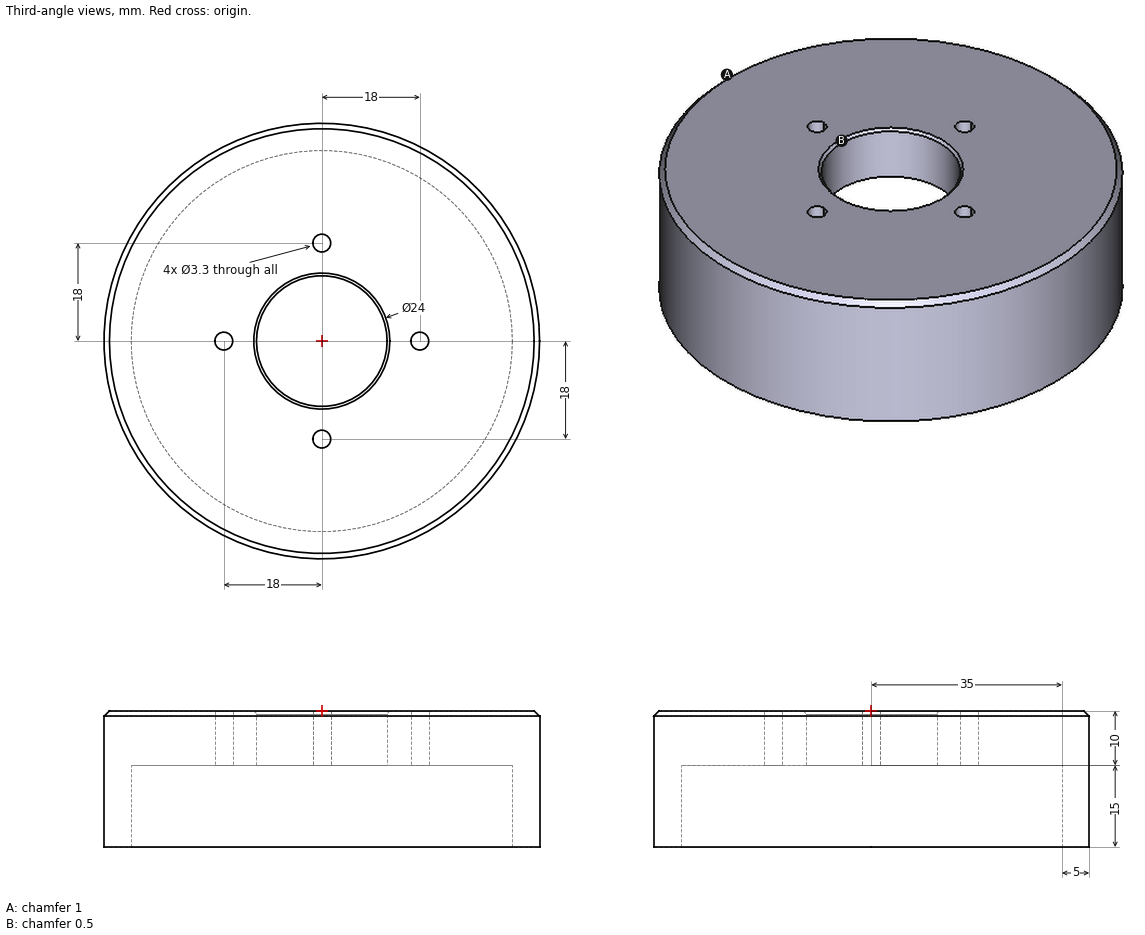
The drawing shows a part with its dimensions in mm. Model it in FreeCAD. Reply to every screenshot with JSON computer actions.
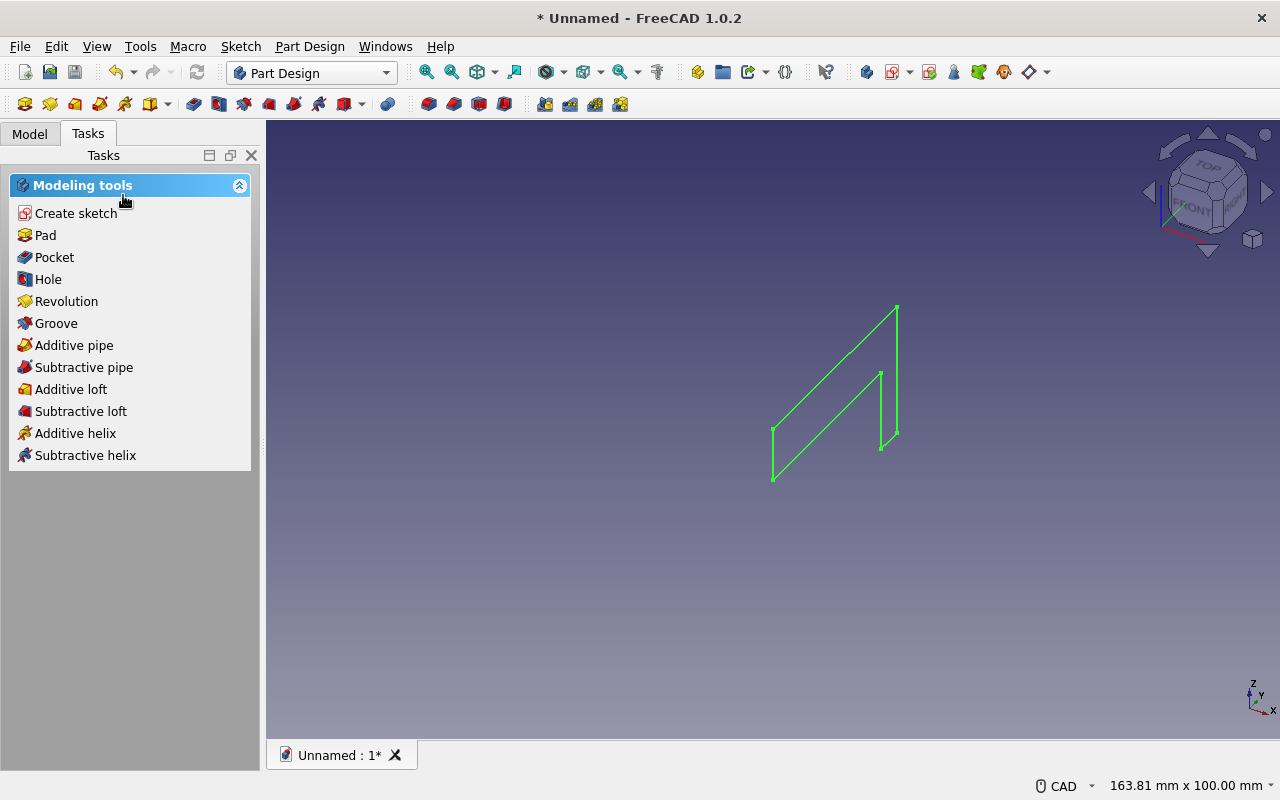
{"action": "left_click", "coordinate": [50, 104]}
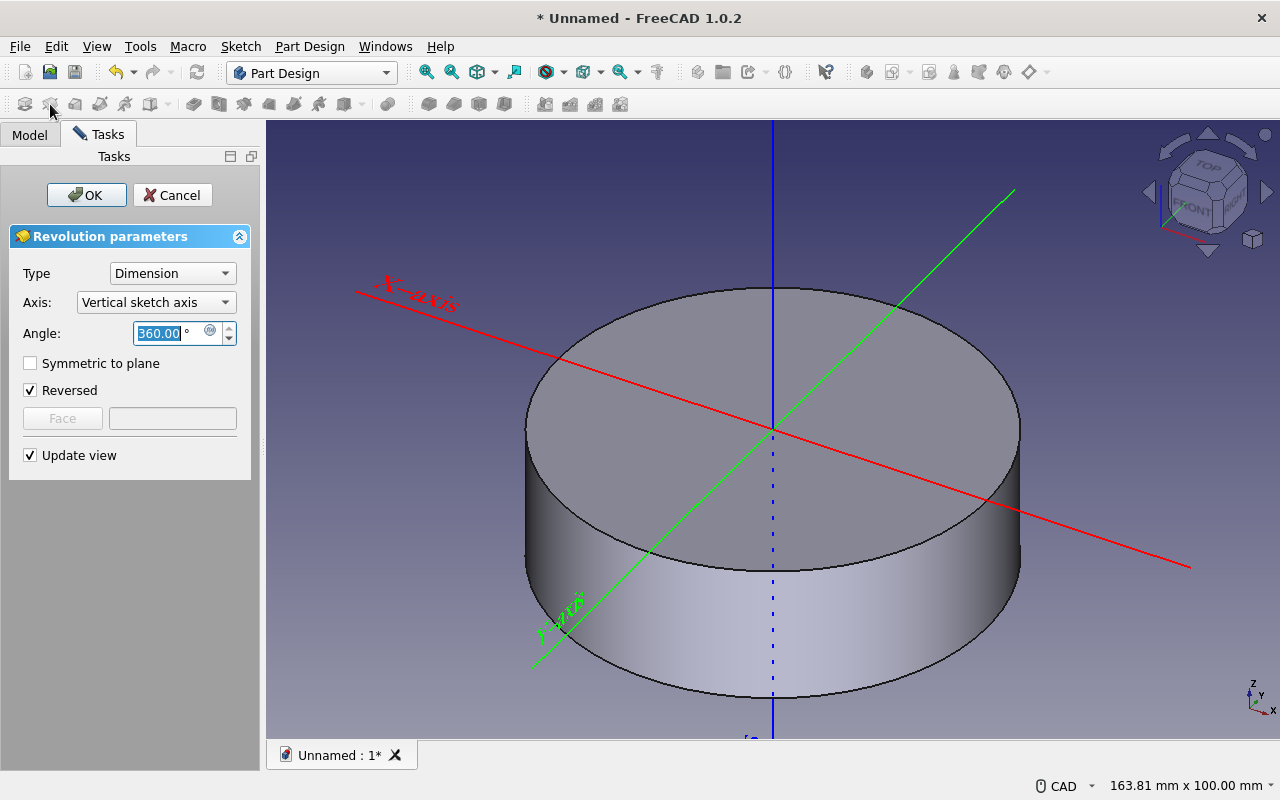
{"action": "left_click", "coordinate": [87, 195]}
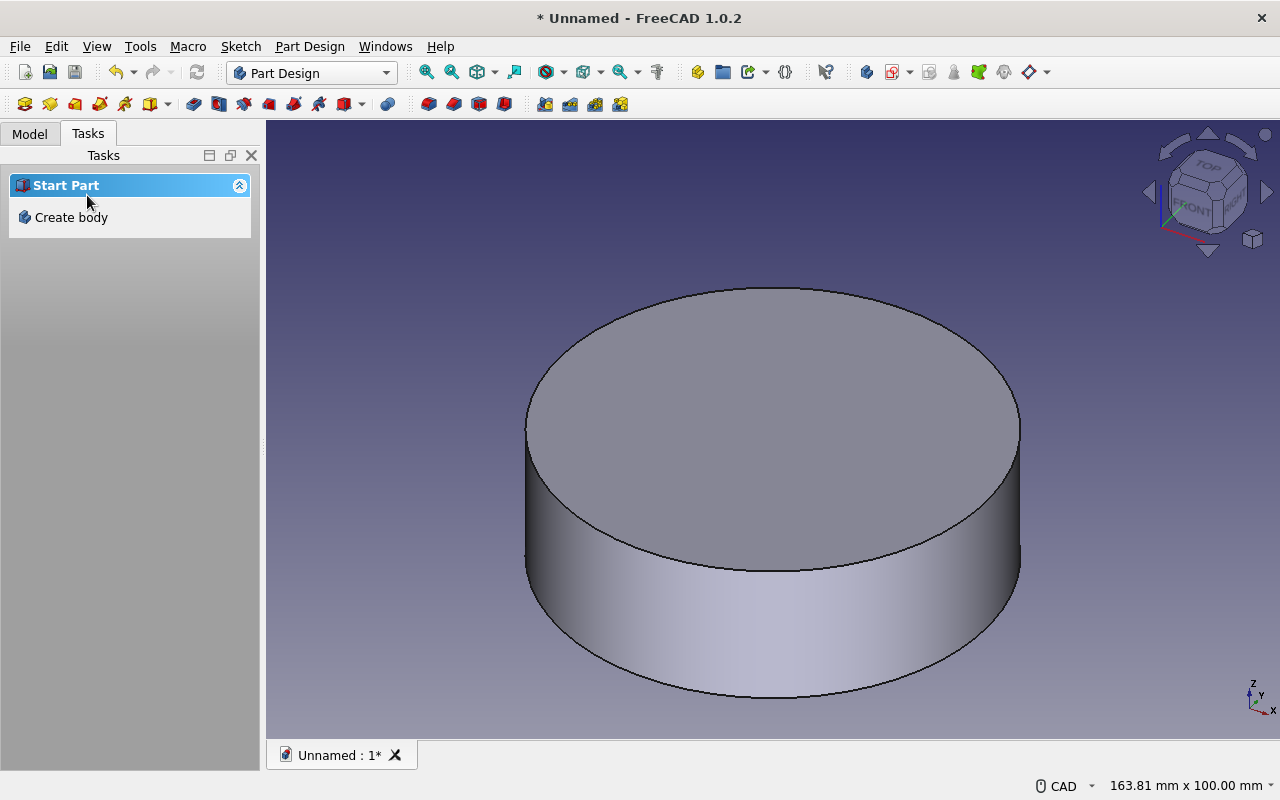
{"action": "key", "text": "v f"}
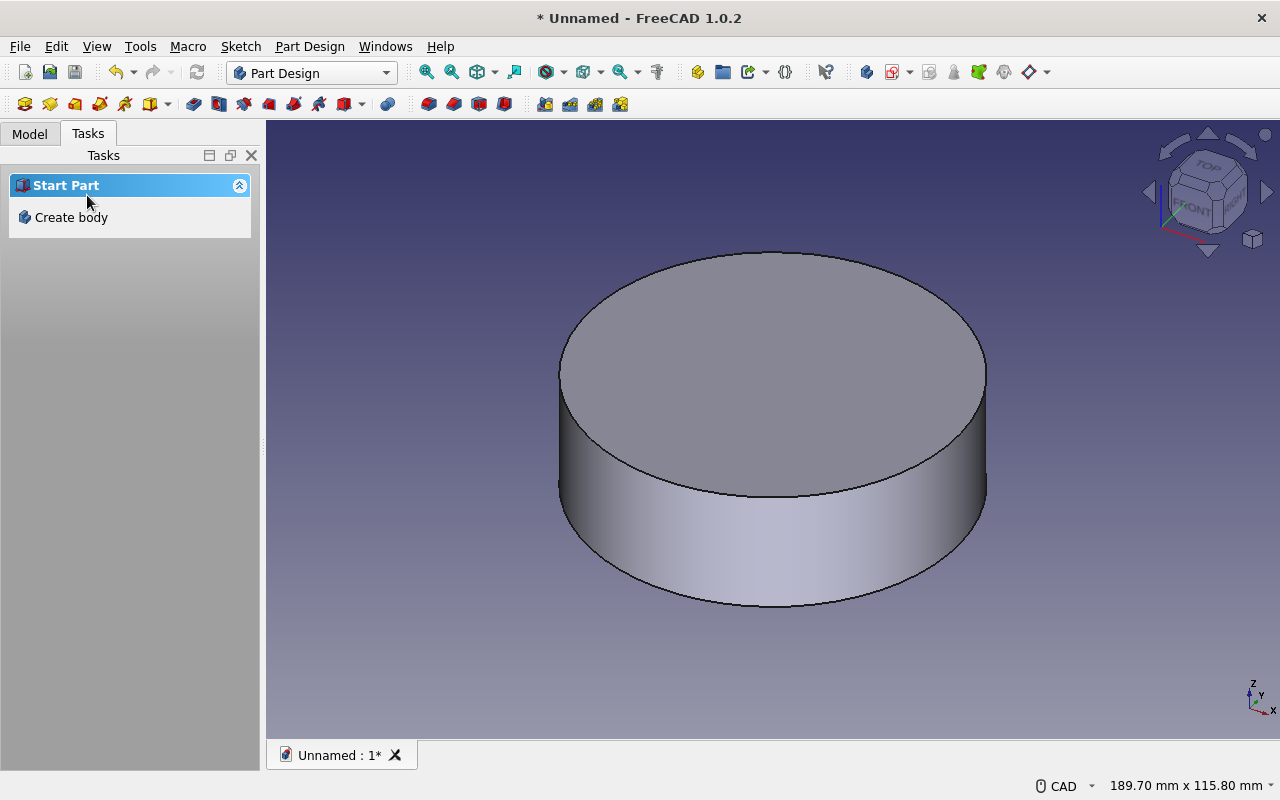
{"action": "left_click", "coordinate": [666, 480]}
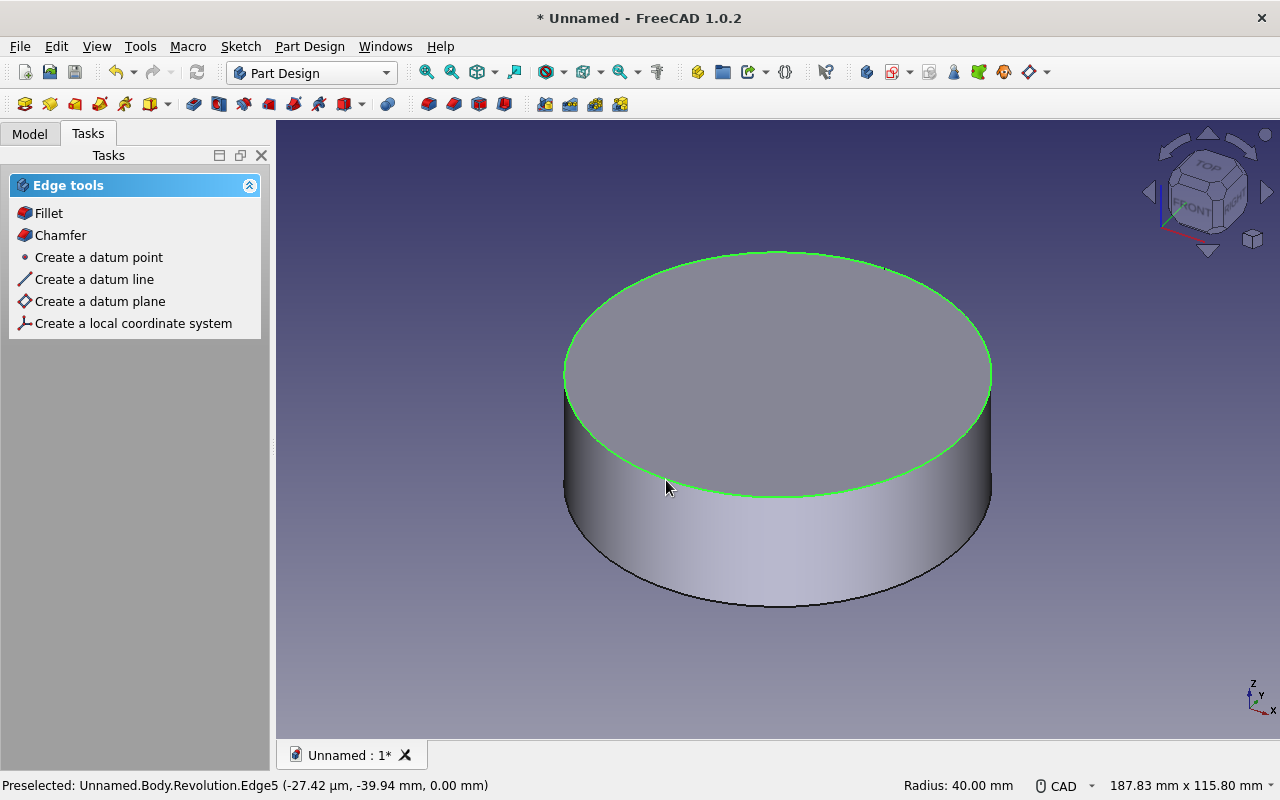
{"action": "left_click", "coordinate": [454, 104]}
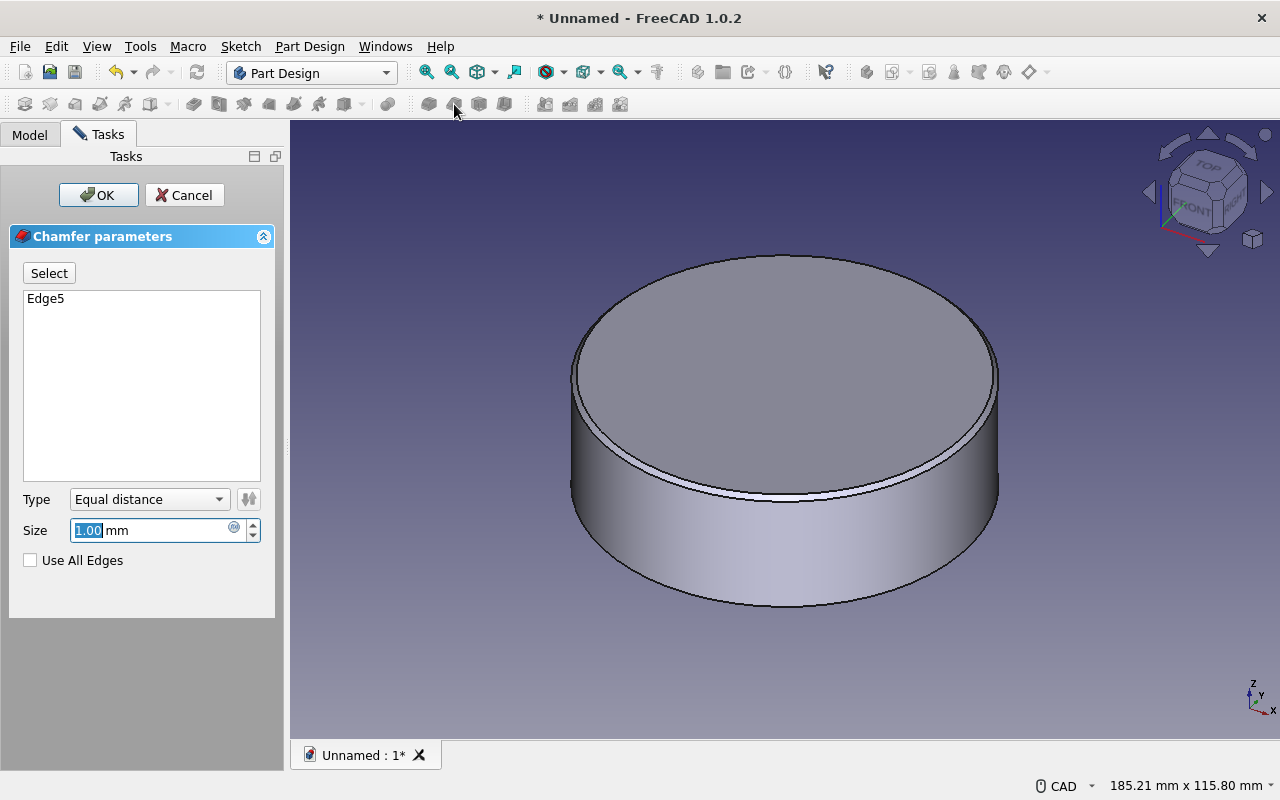
{"action": "type", "text": "1"}
{"action": "key", "text": "Tab"}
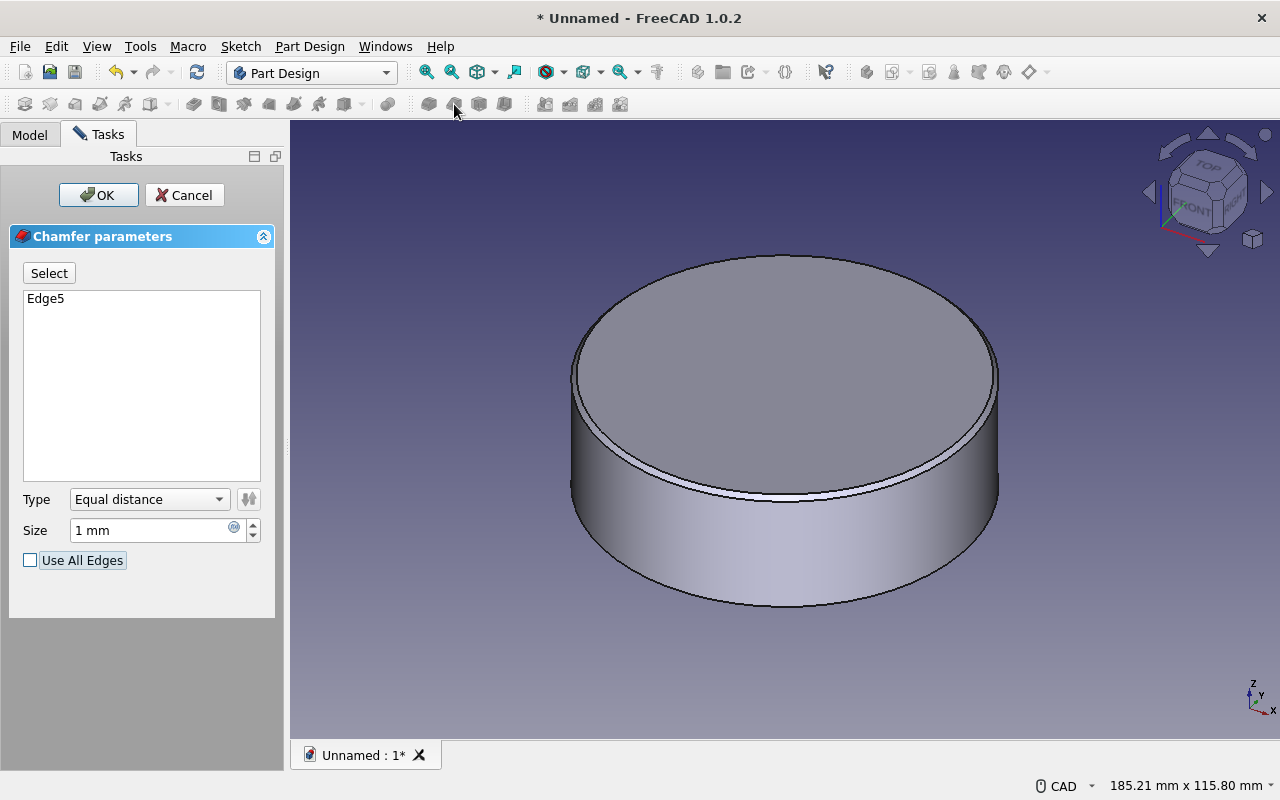
{"action": "left_click", "coordinate": [99, 195]}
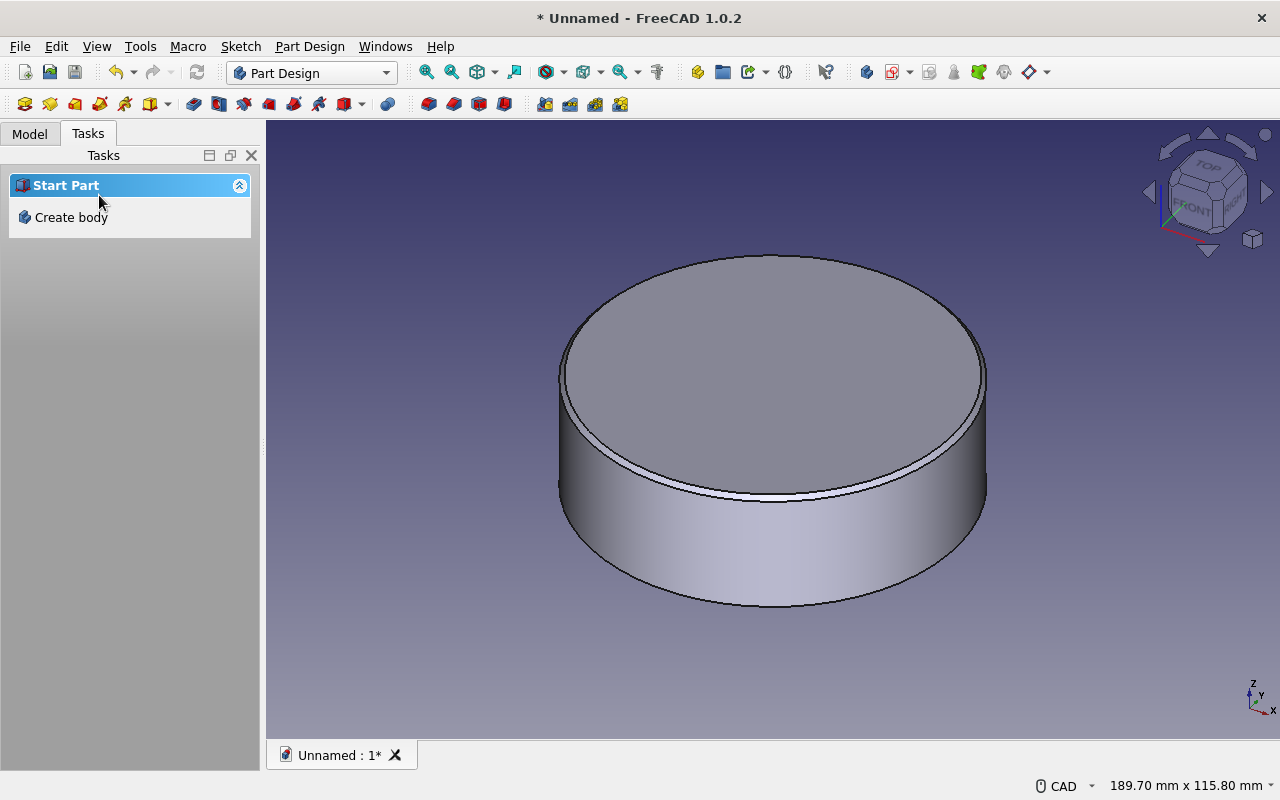
{"action": "left_click", "coordinate": [773, 374]}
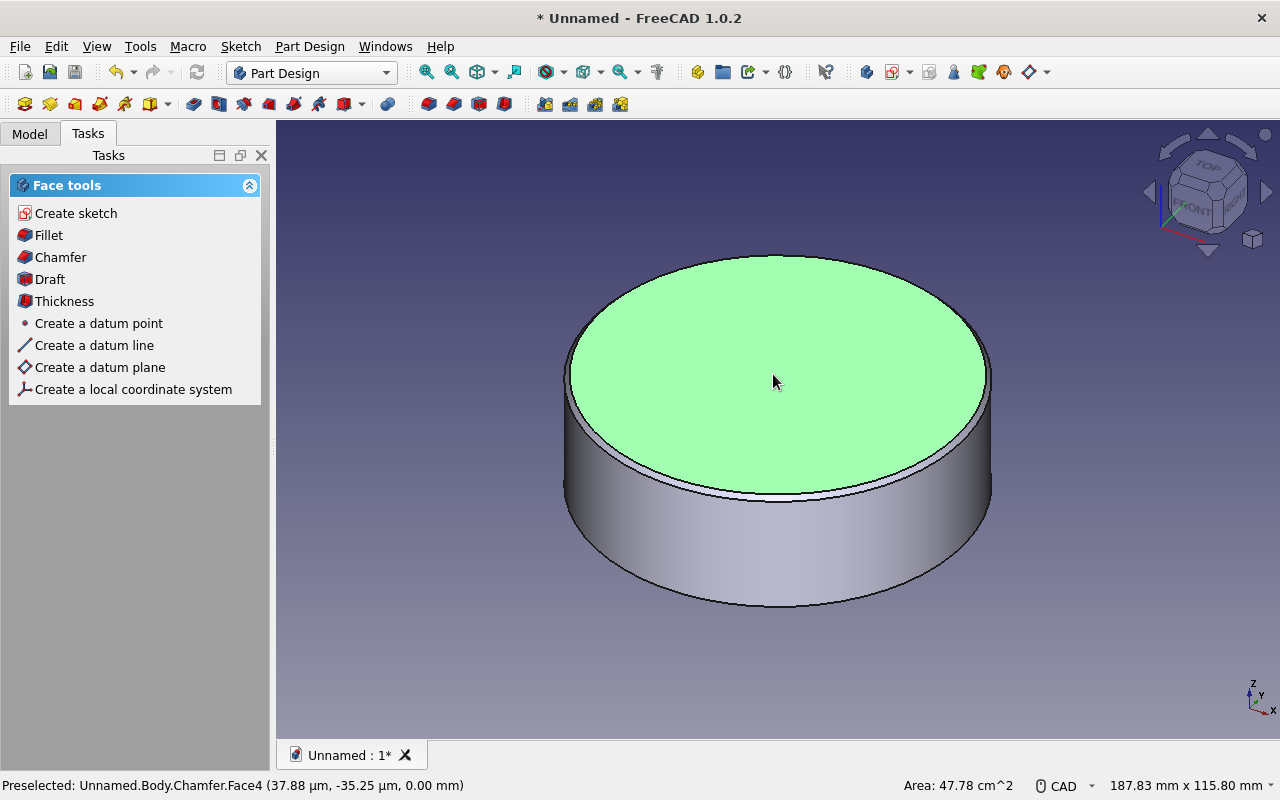
{"action": "left_click", "coordinate": [892, 72]}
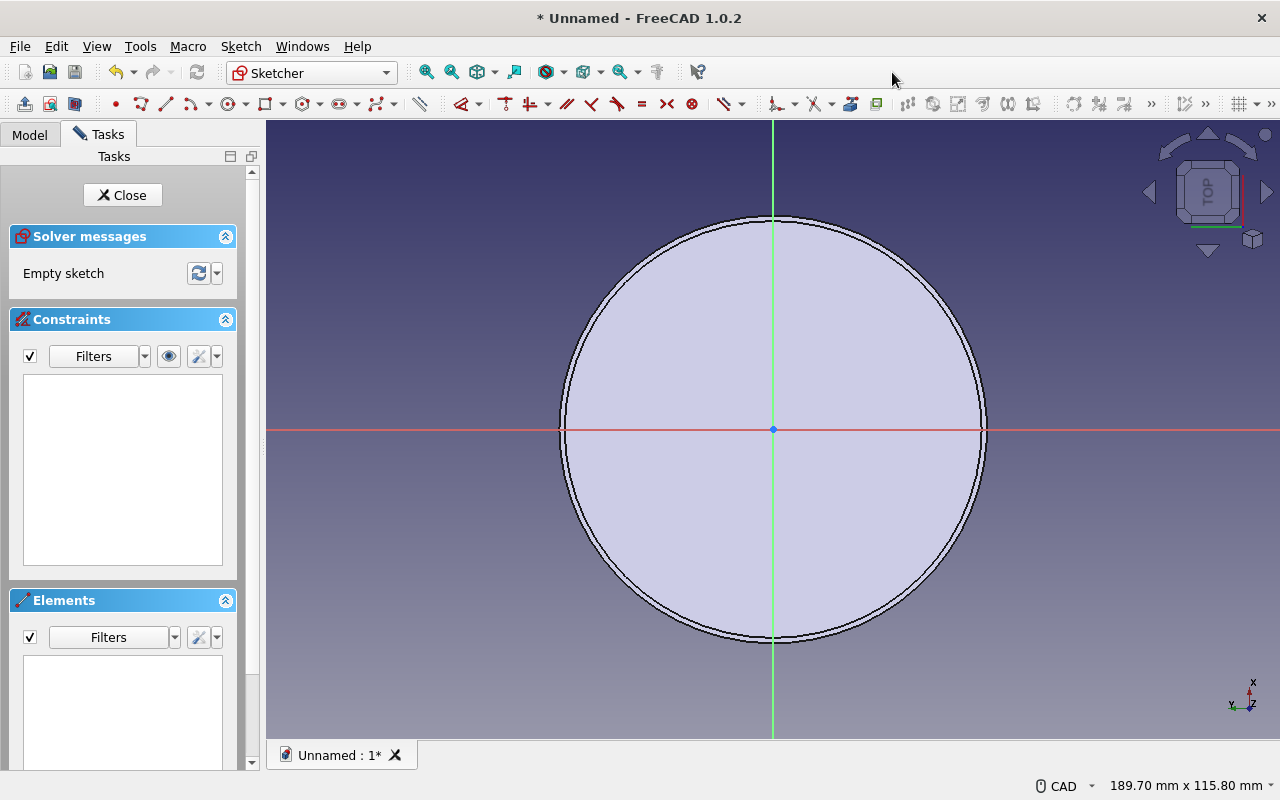
{"action": "scroll", "coordinate": [803, 430], "scroll_direction": "up", "scroll_amount": 6}